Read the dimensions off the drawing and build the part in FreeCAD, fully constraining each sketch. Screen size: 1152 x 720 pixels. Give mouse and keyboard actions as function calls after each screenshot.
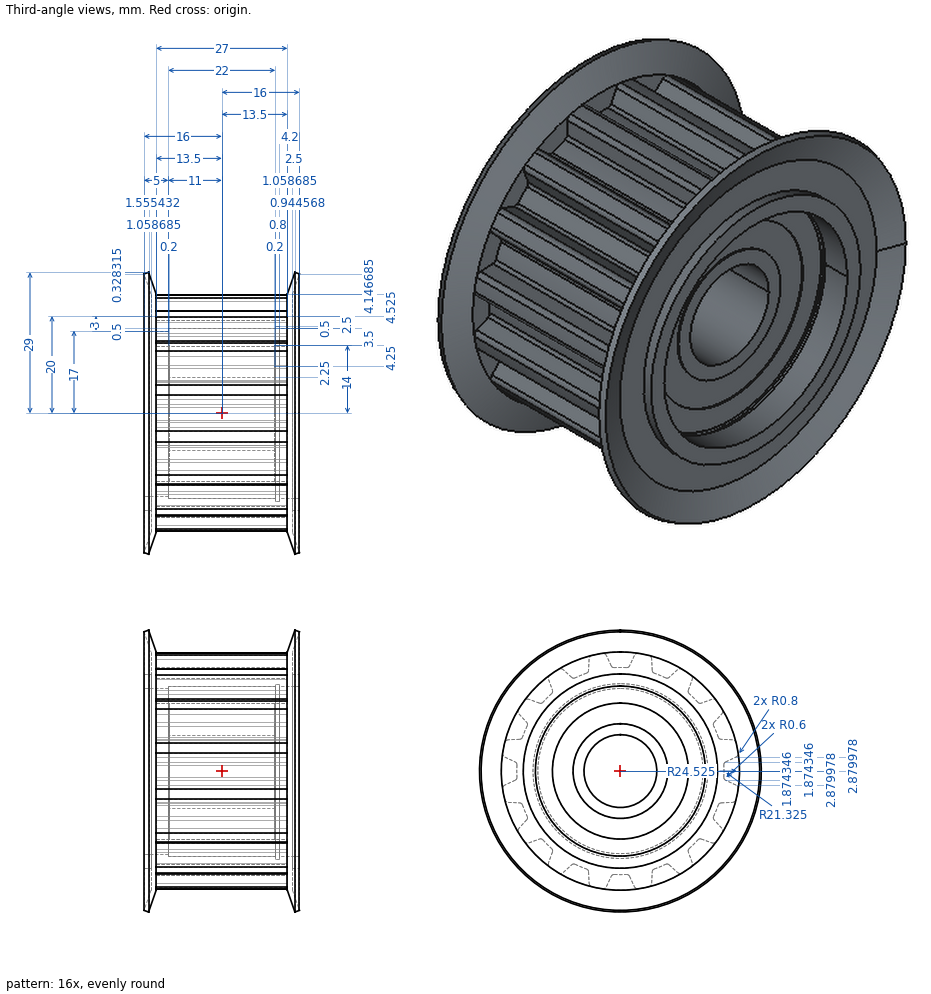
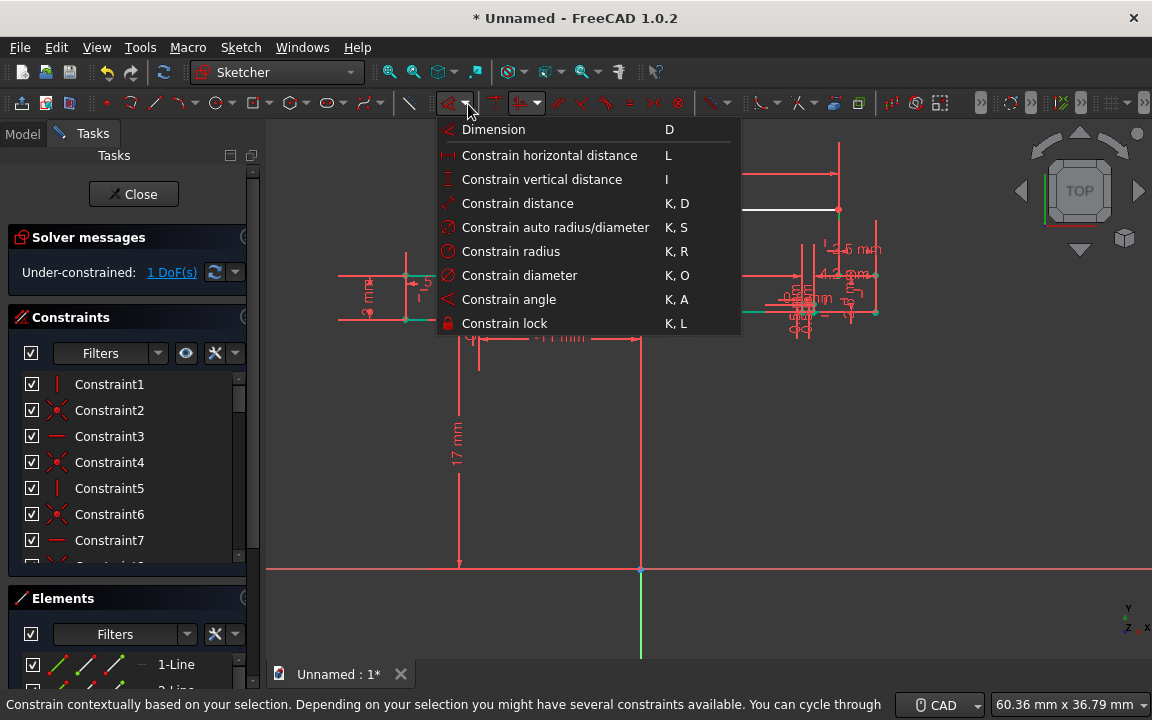
click(589, 179)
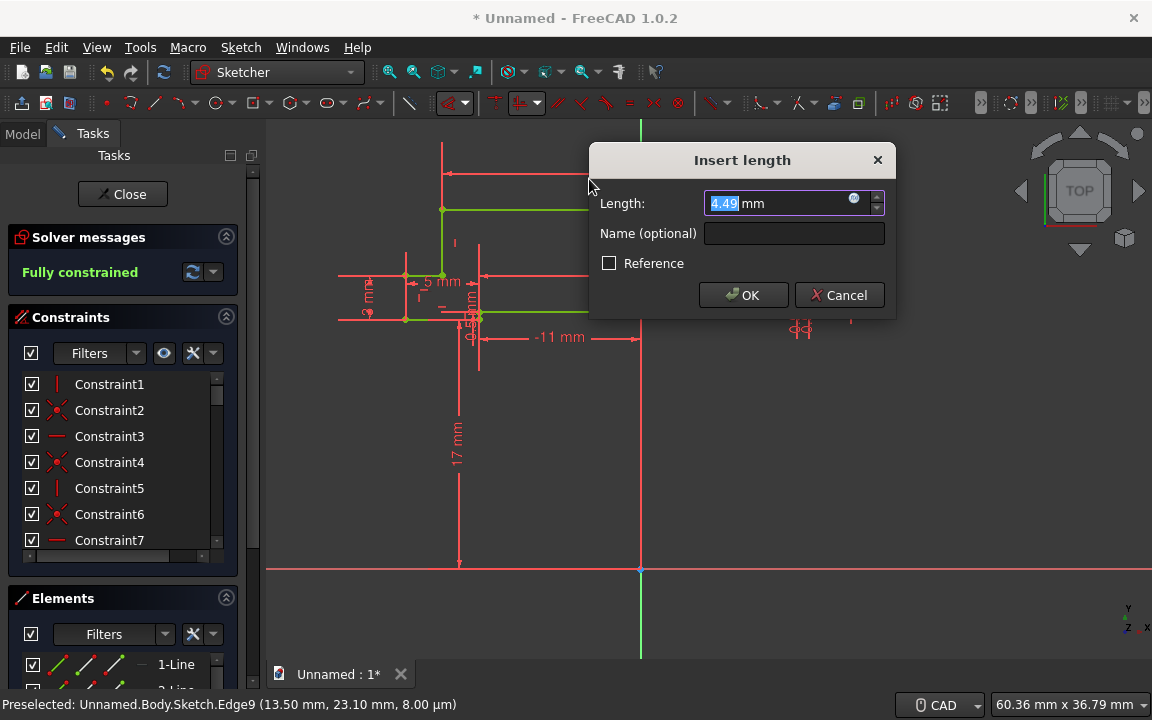
text(4.525)
key(Return)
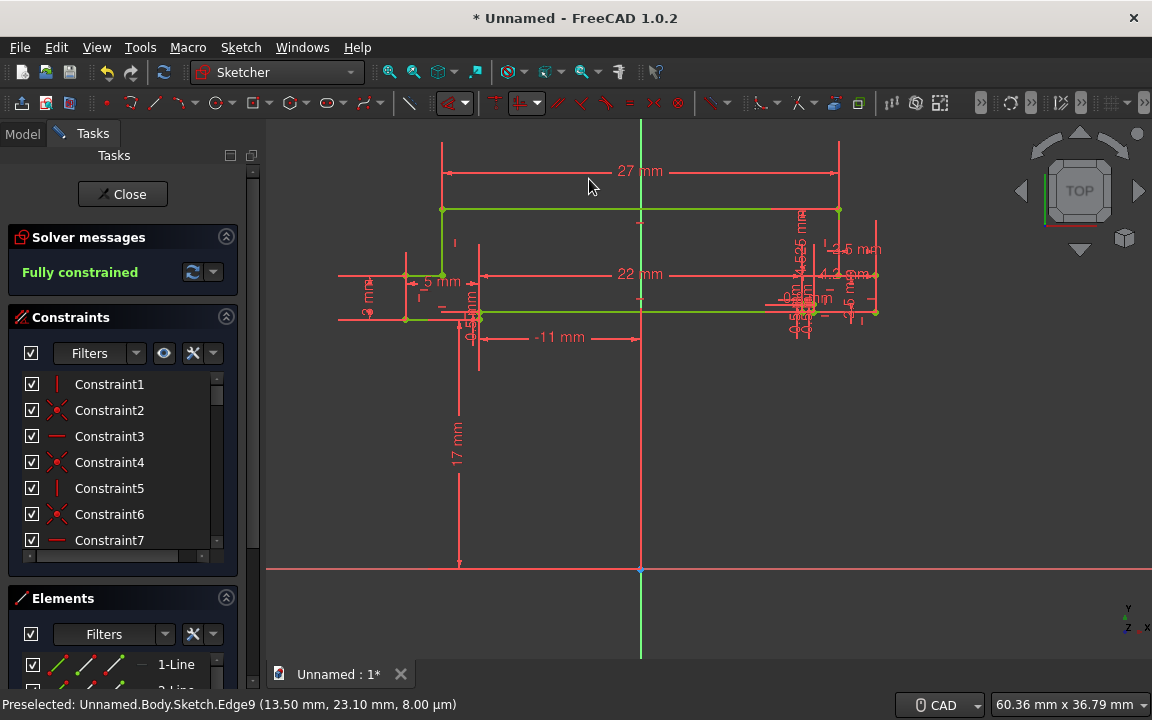
click(123, 194)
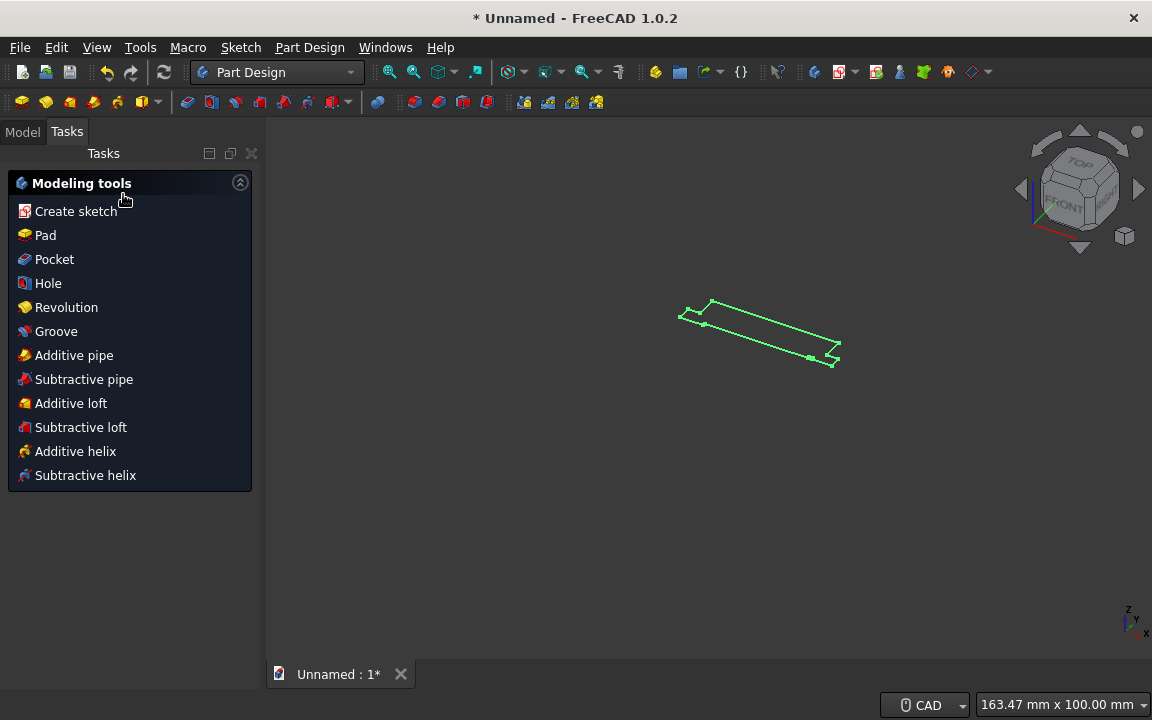
click(46, 102)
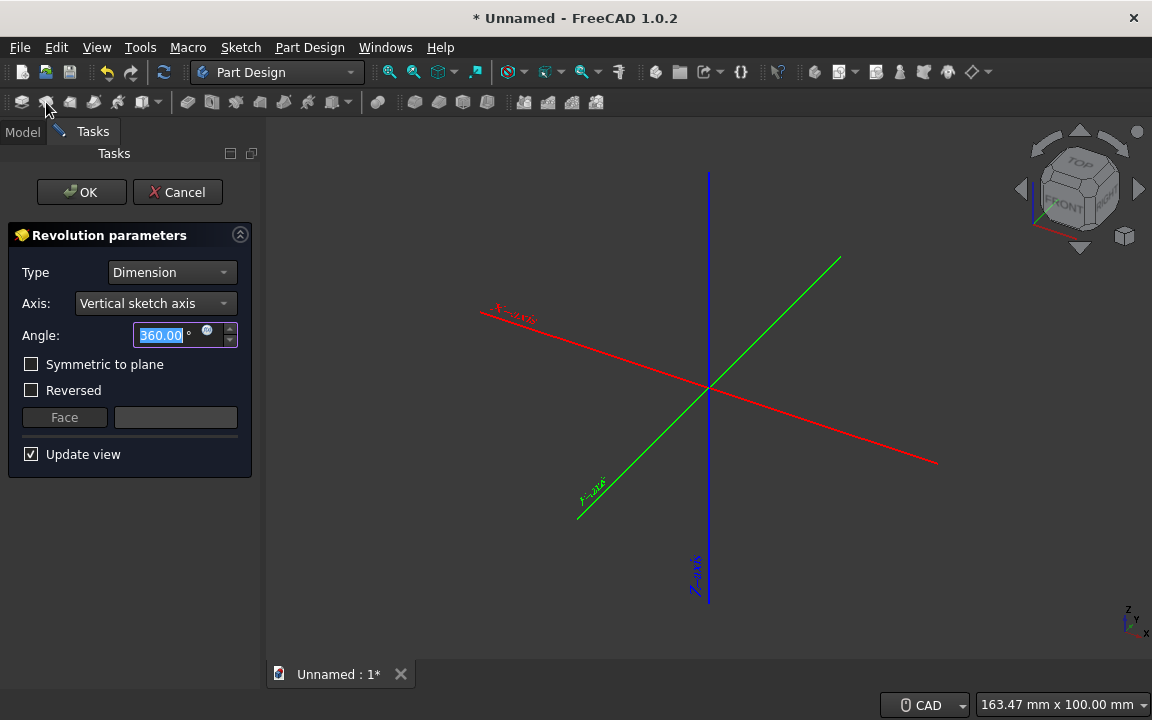
click(156, 304)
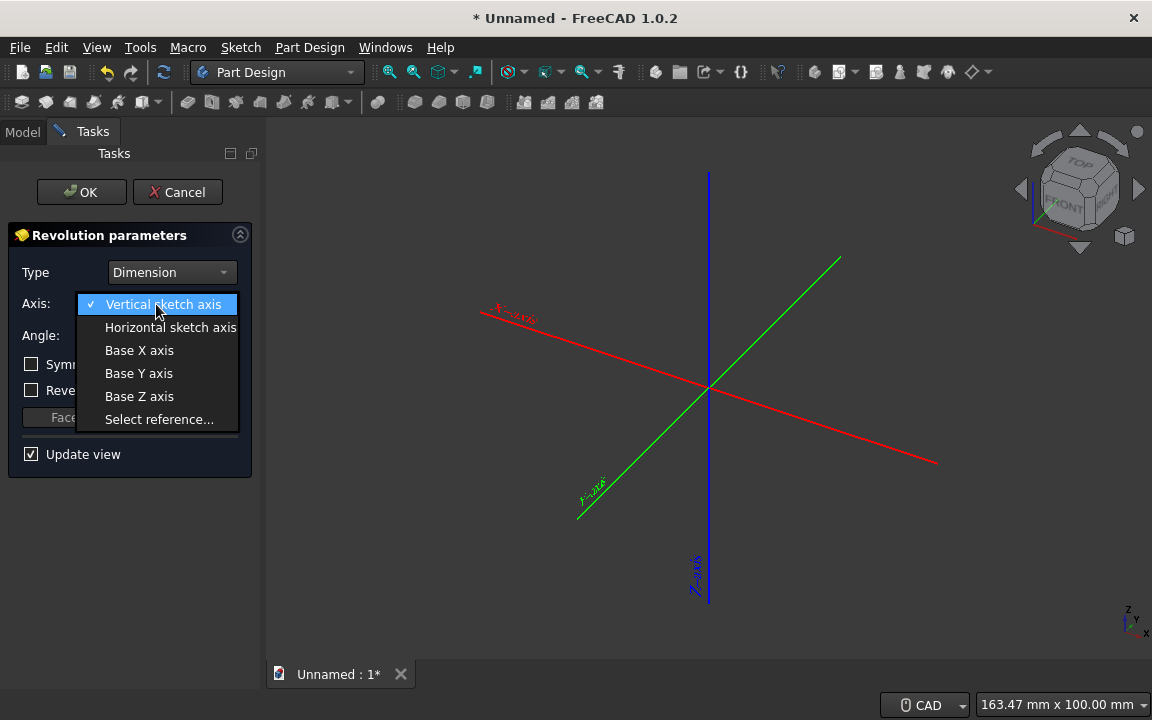
click(156, 328)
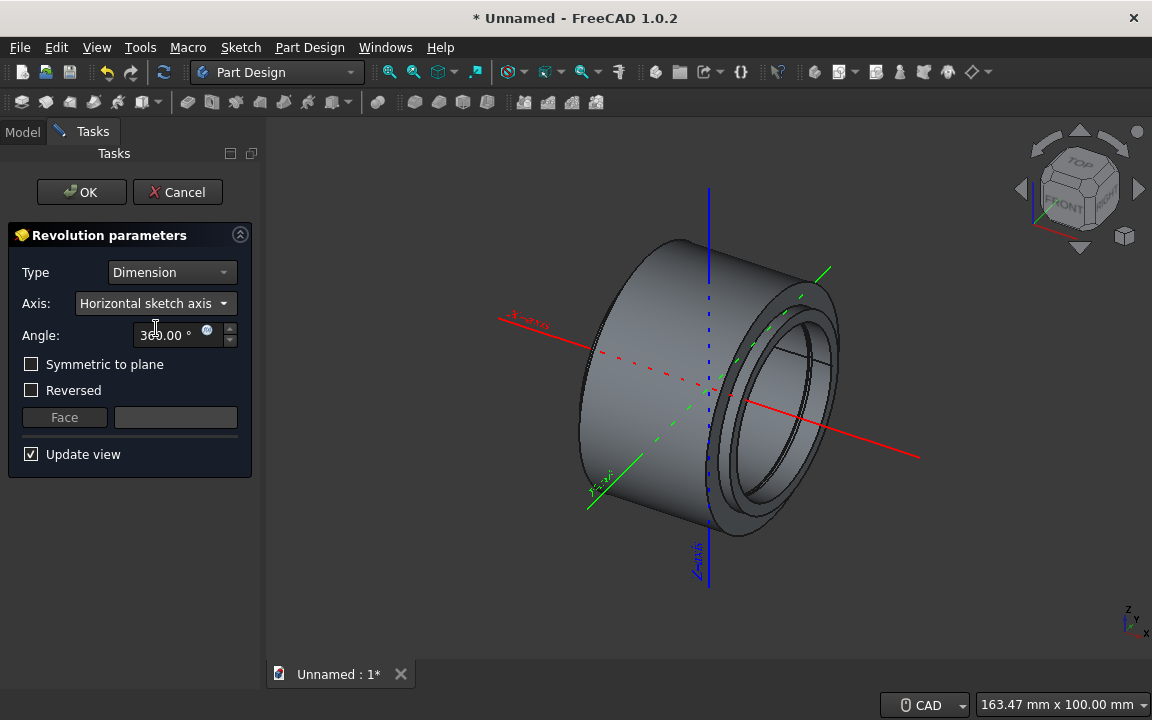
click(82, 192)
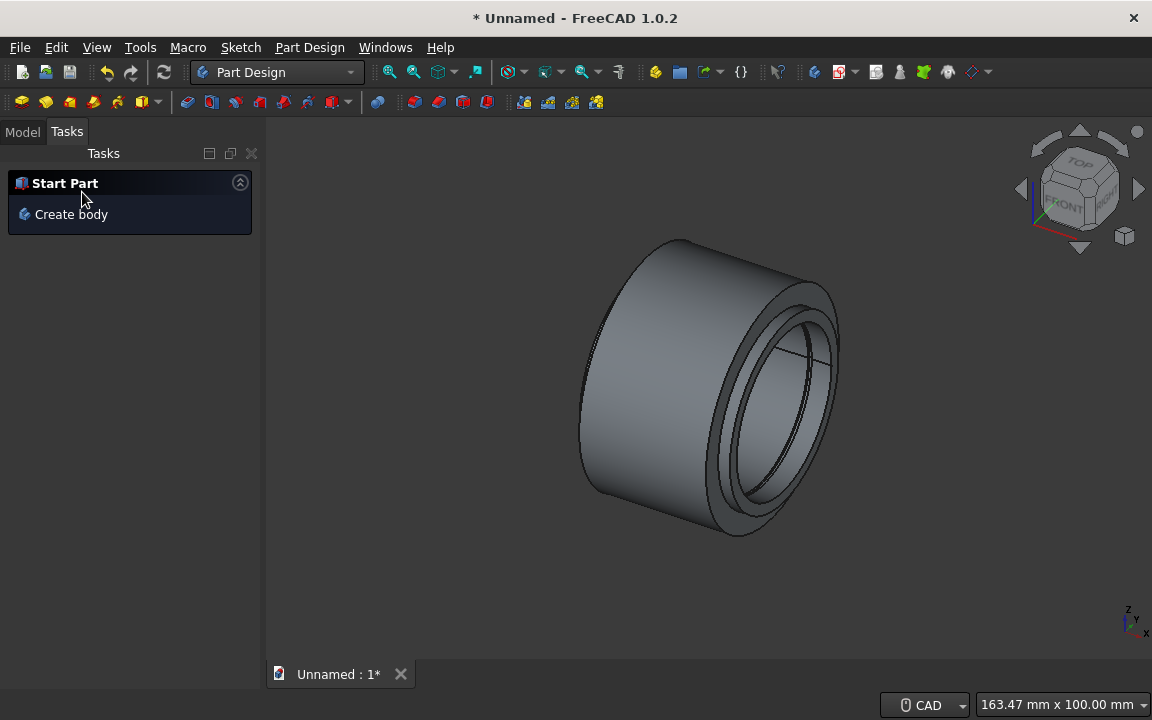
click(23, 131)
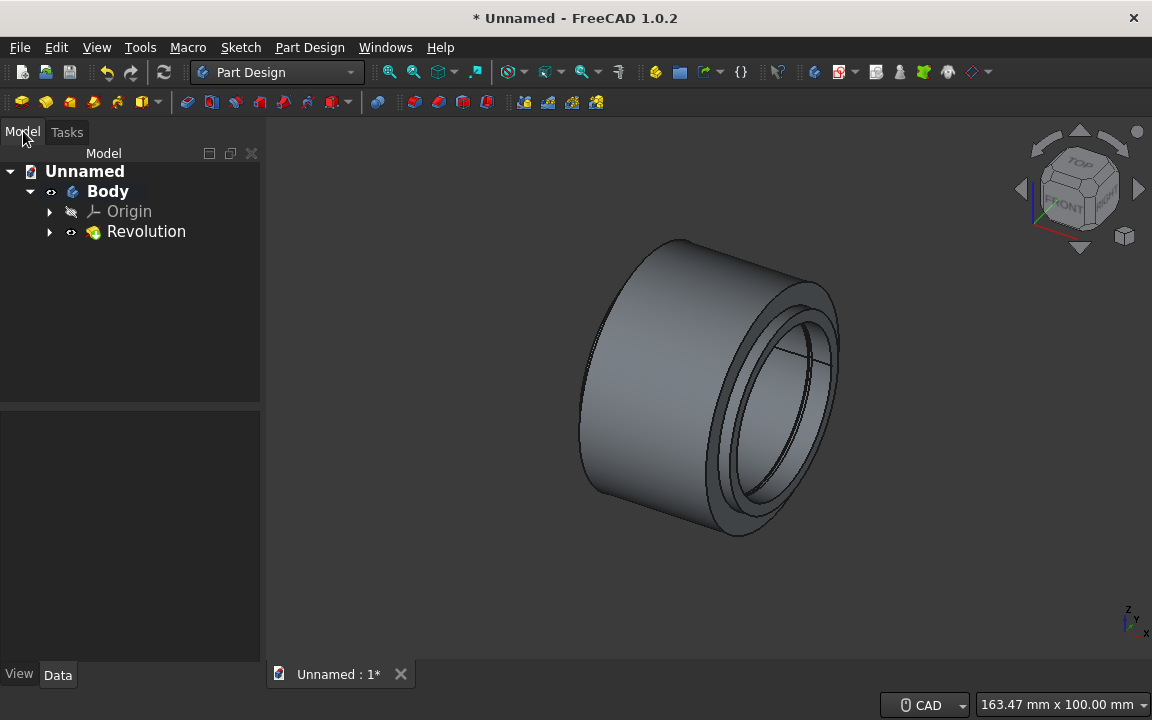
click(50, 212)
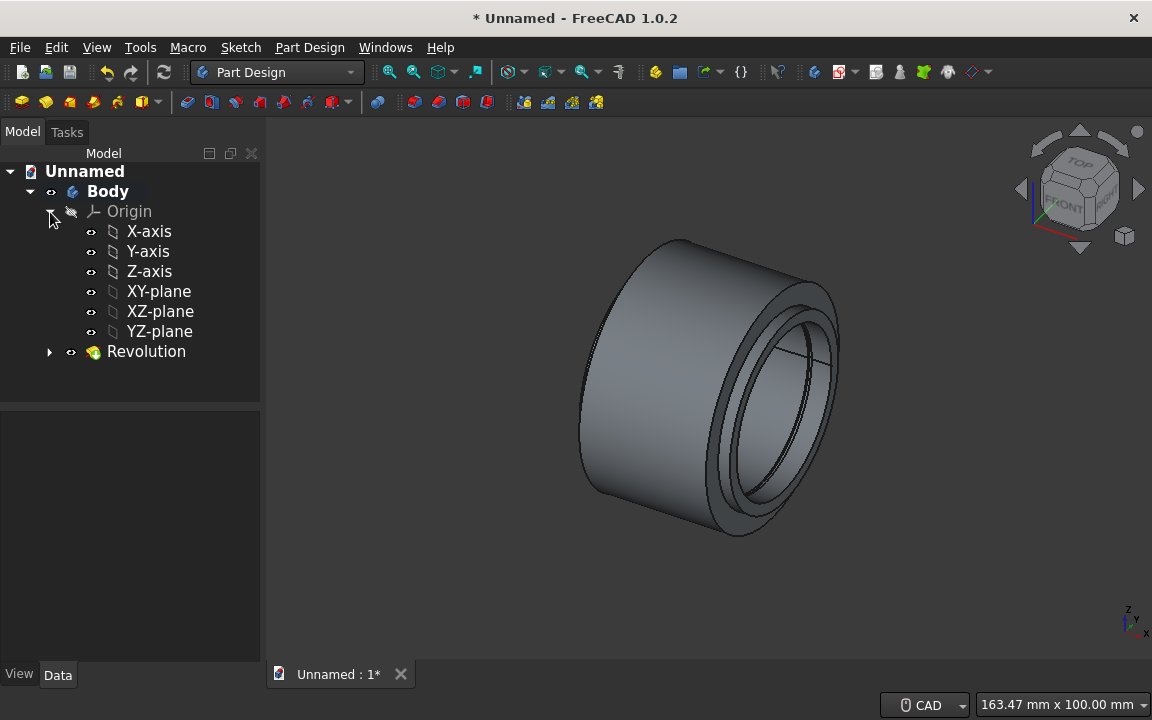
click(136, 332)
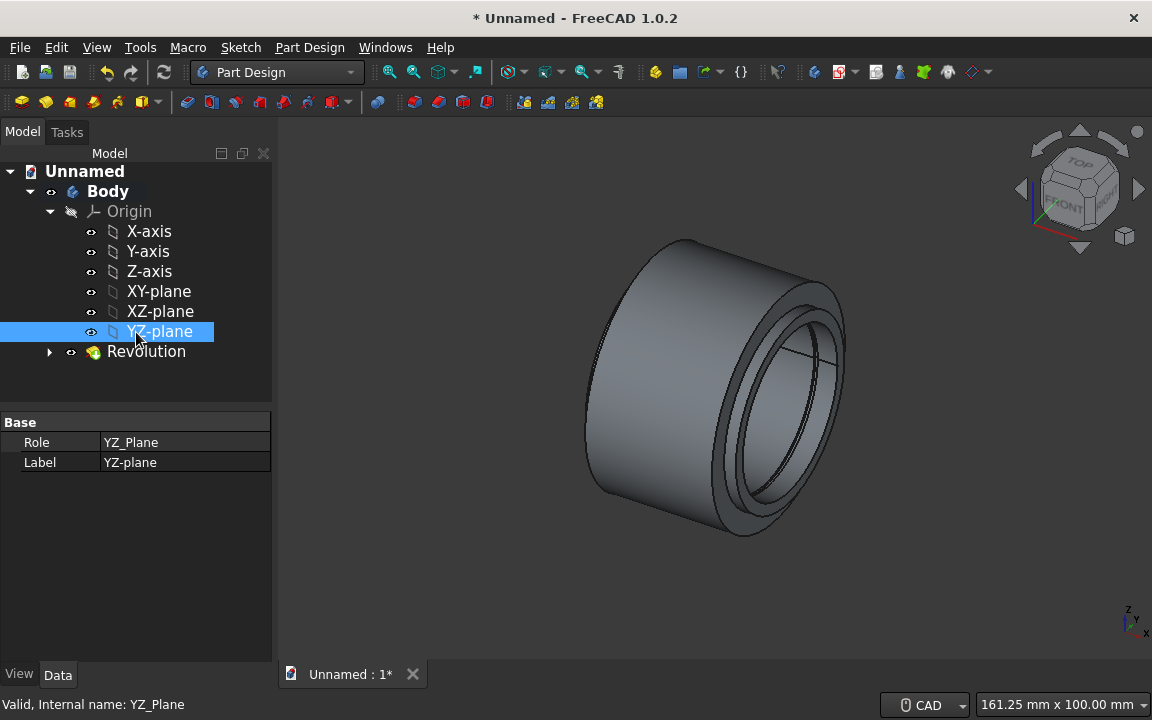
click(972, 72)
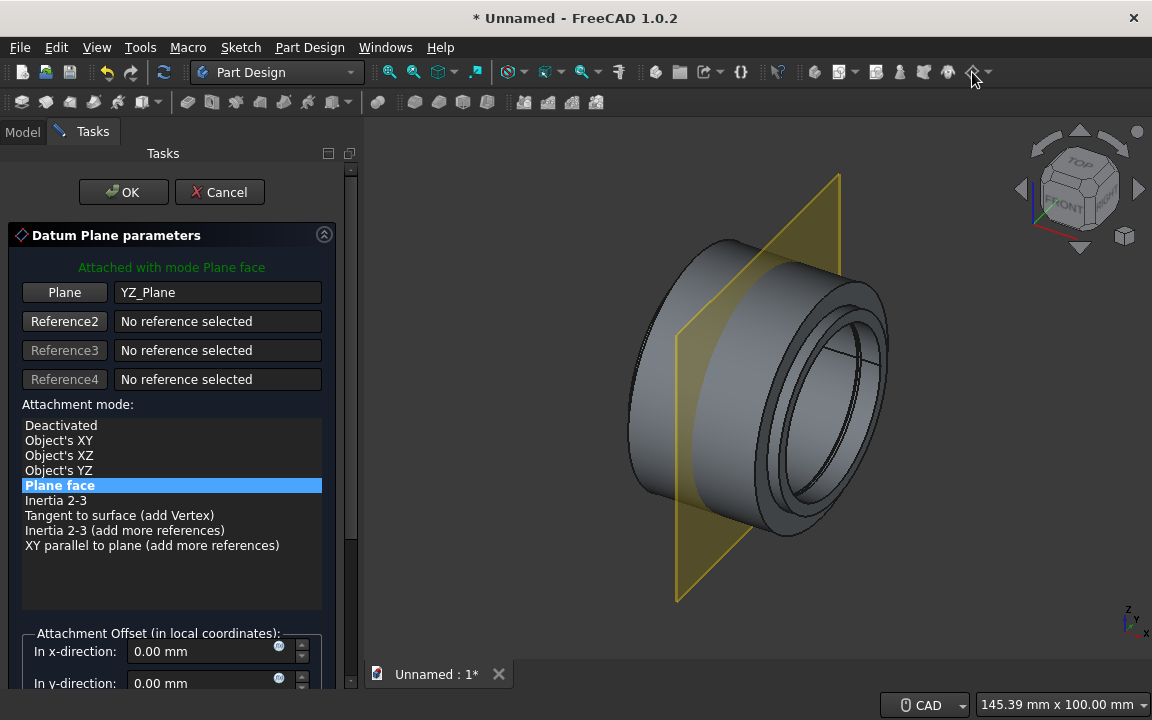
scroll(351, 426, down, 2)